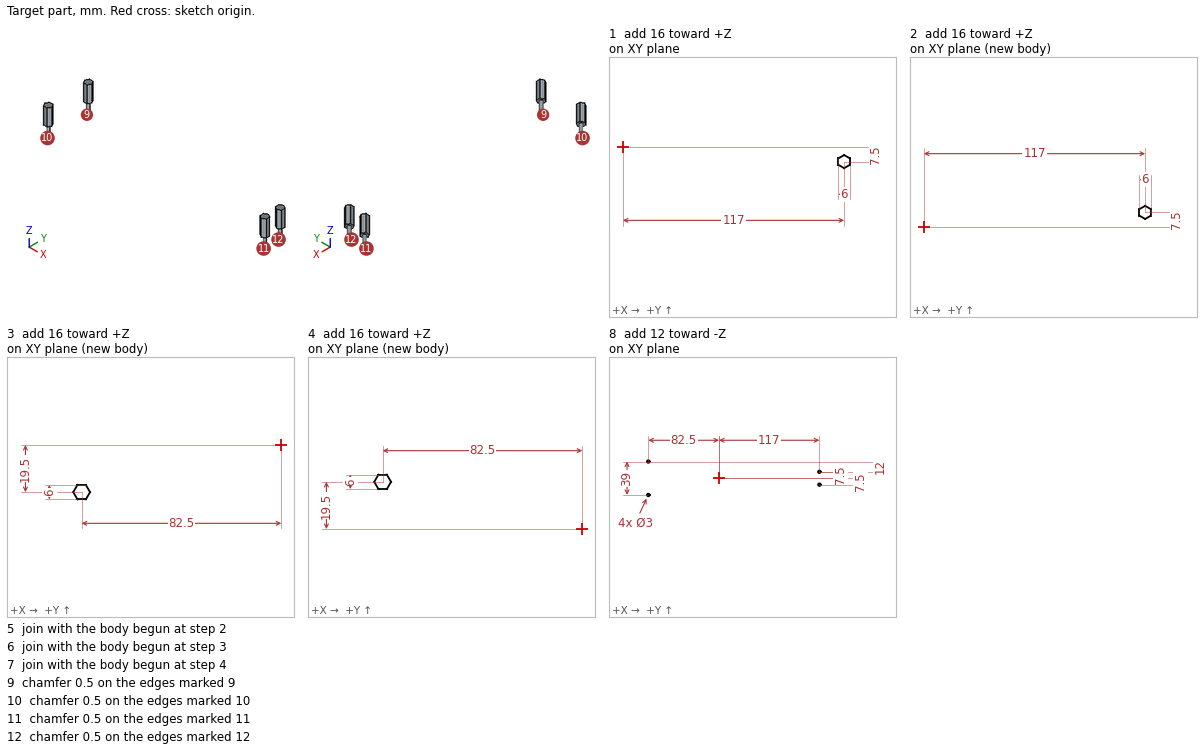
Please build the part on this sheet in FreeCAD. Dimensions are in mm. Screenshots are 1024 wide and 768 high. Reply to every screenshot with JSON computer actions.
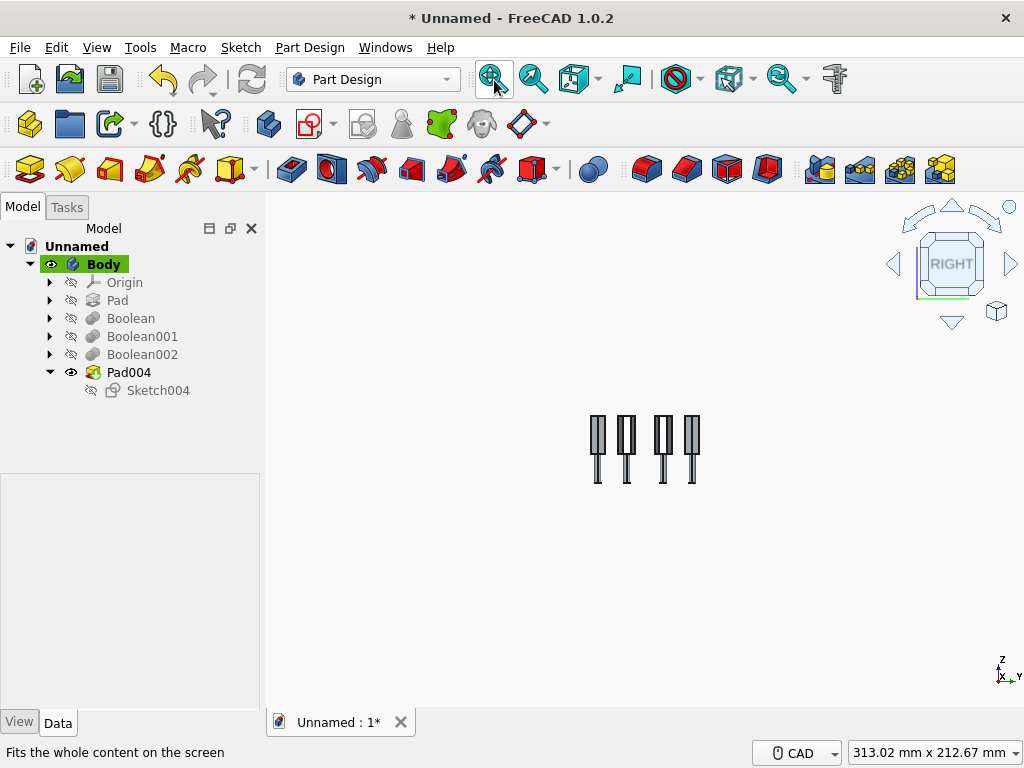
{"action": "left_click", "coordinate": [494, 80]}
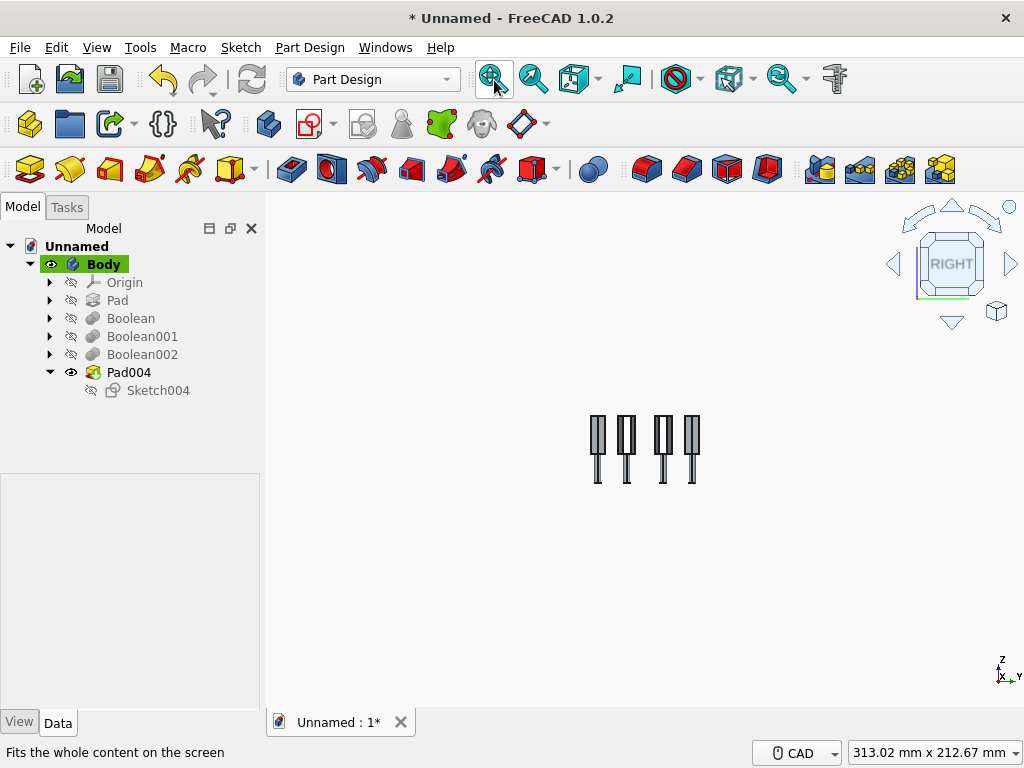
{"action": "key", "text": "5"}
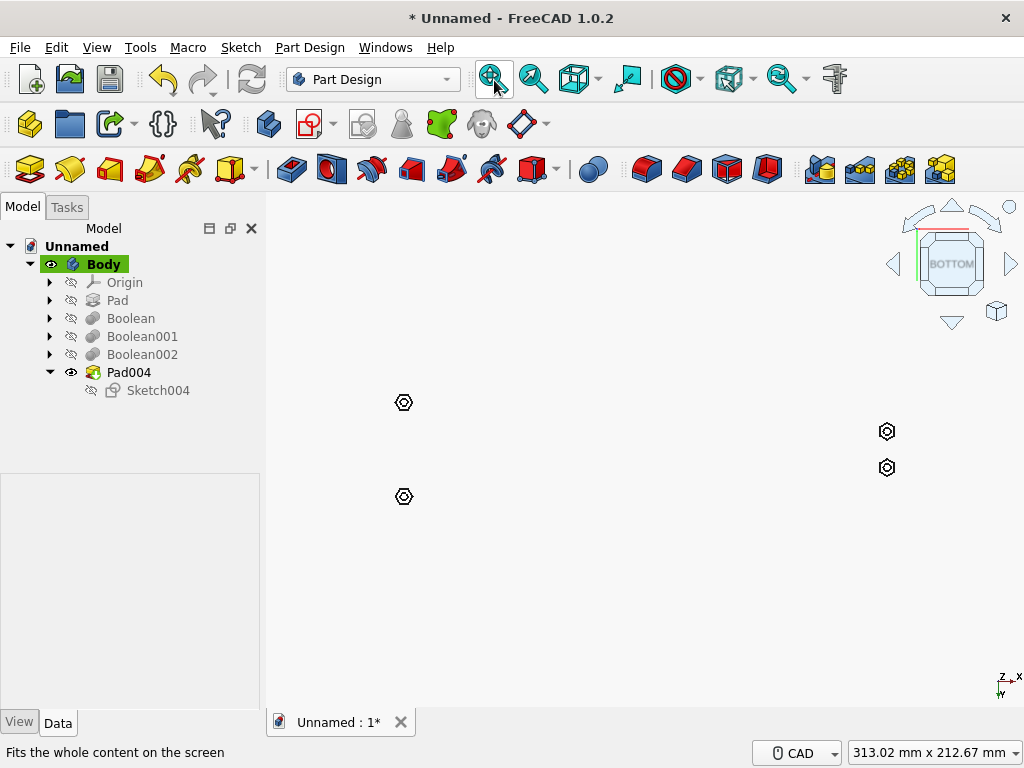
{"action": "left_click", "coordinate": [400, 496]}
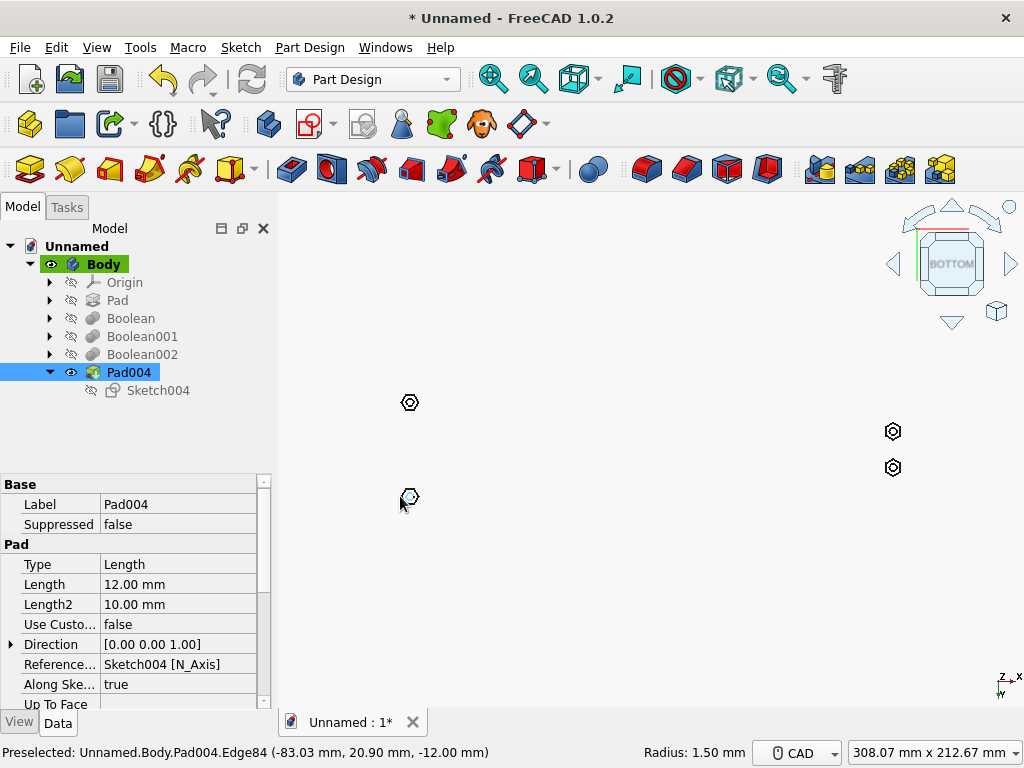
{"action": "left_click", "coordinate": [688, 170]}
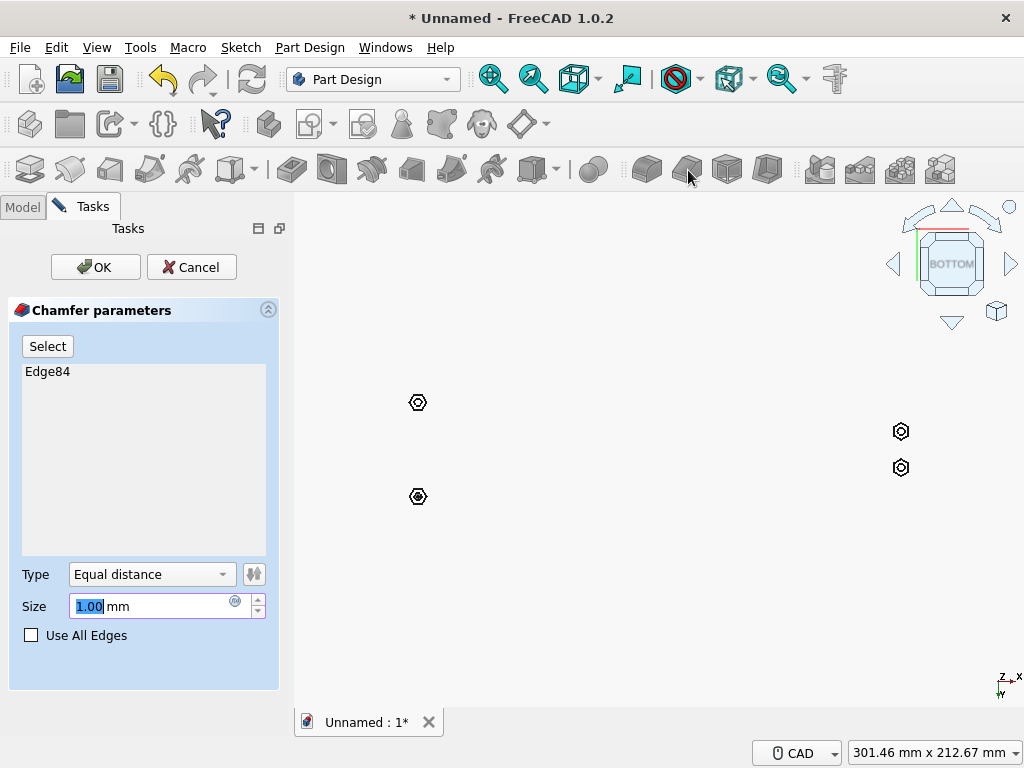
{"action": "type", "text": "0.5"}
{"action": "key", "text": "Tab"}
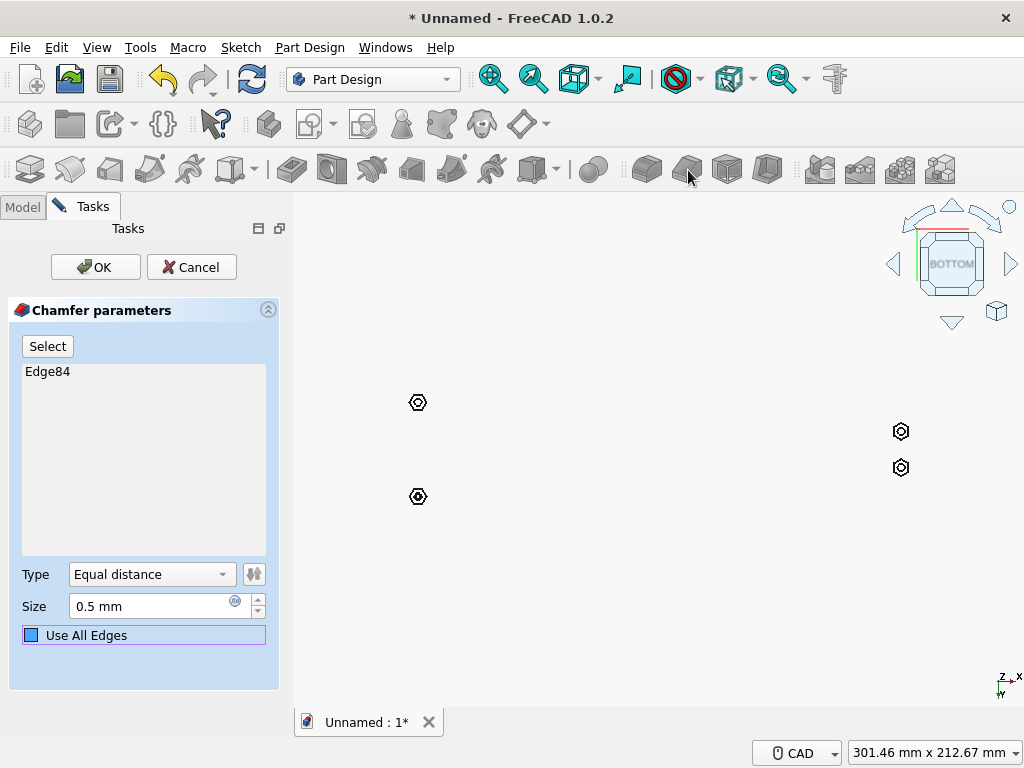
{"action": "left_click", "coordinate": [96, 267]}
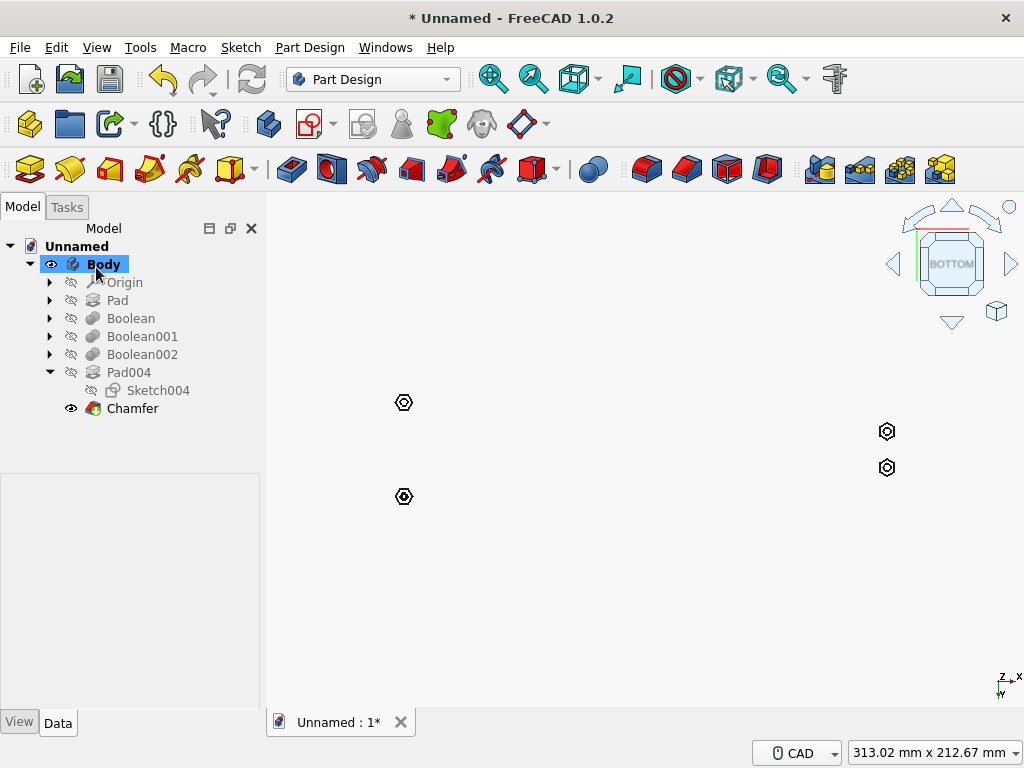
{"action": "left_click", "coordinate": [400, 401]}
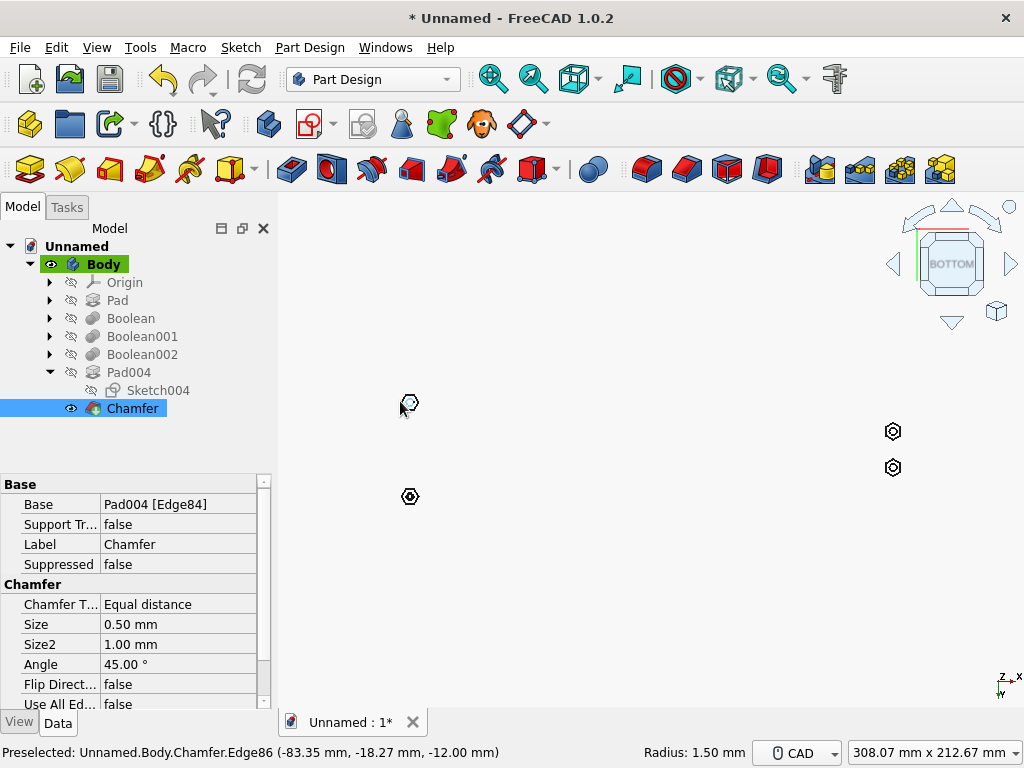
{"action": "left_click", "coordinate": [688, 170]}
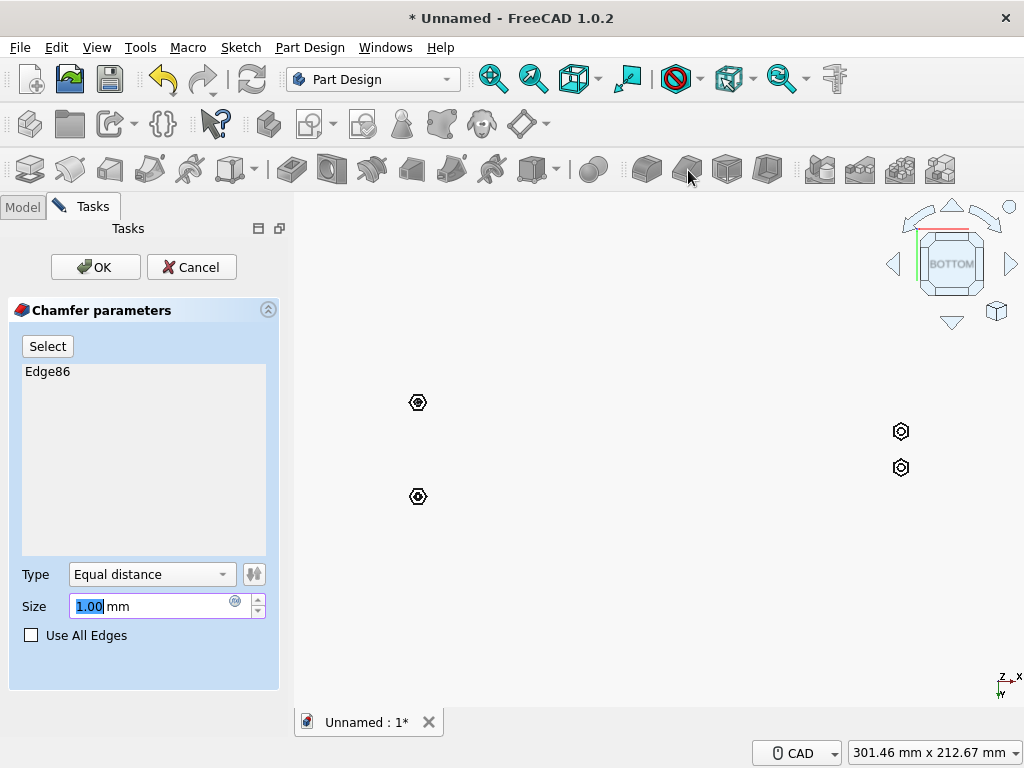
{"action": "type", "text": "0.5"}
{"action": "key", "text": "Tab"}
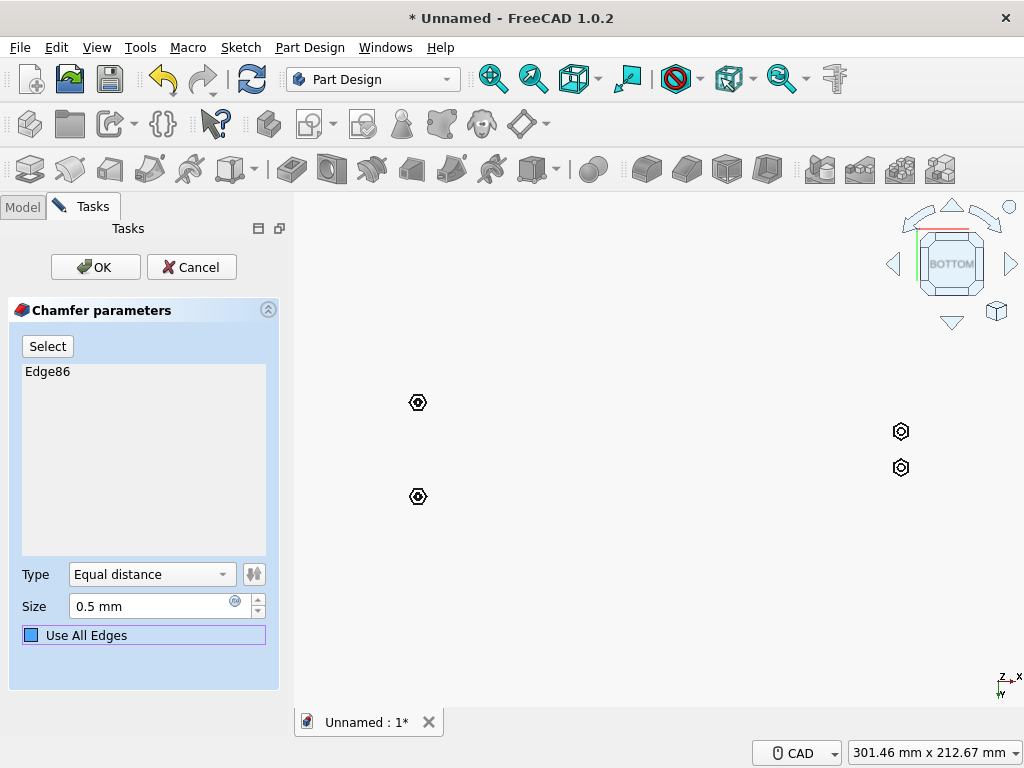
{"action": "left_click", "coordinate": [96, 267]}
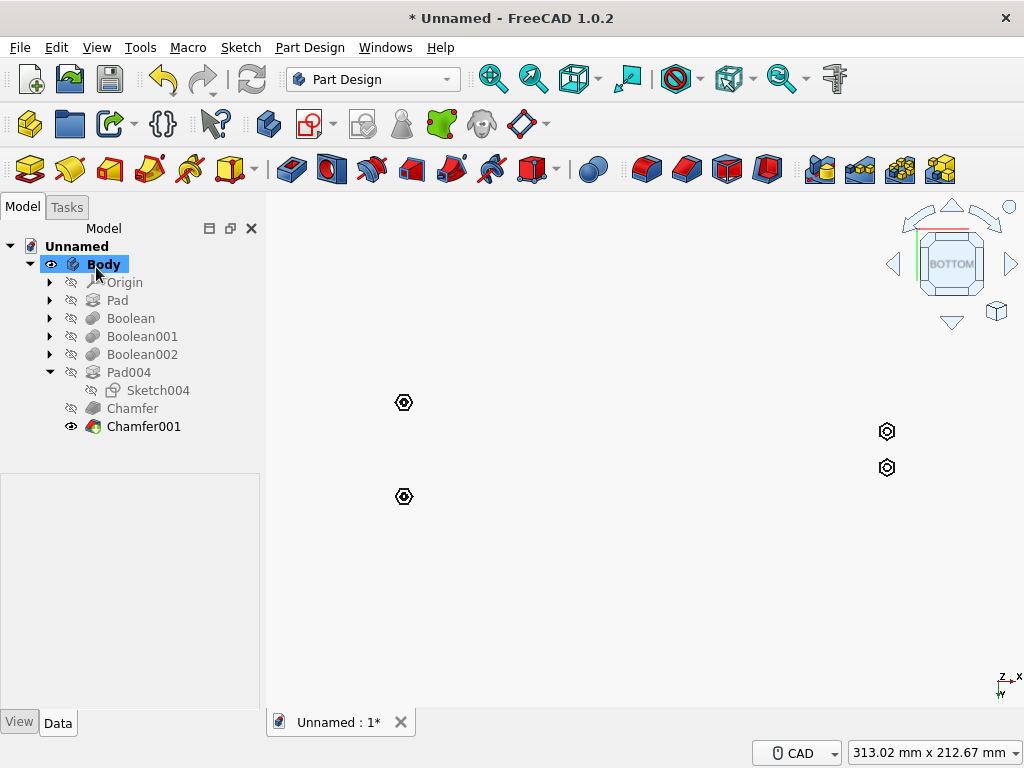
{"action": "left_click", "coordinate": [883, 430]}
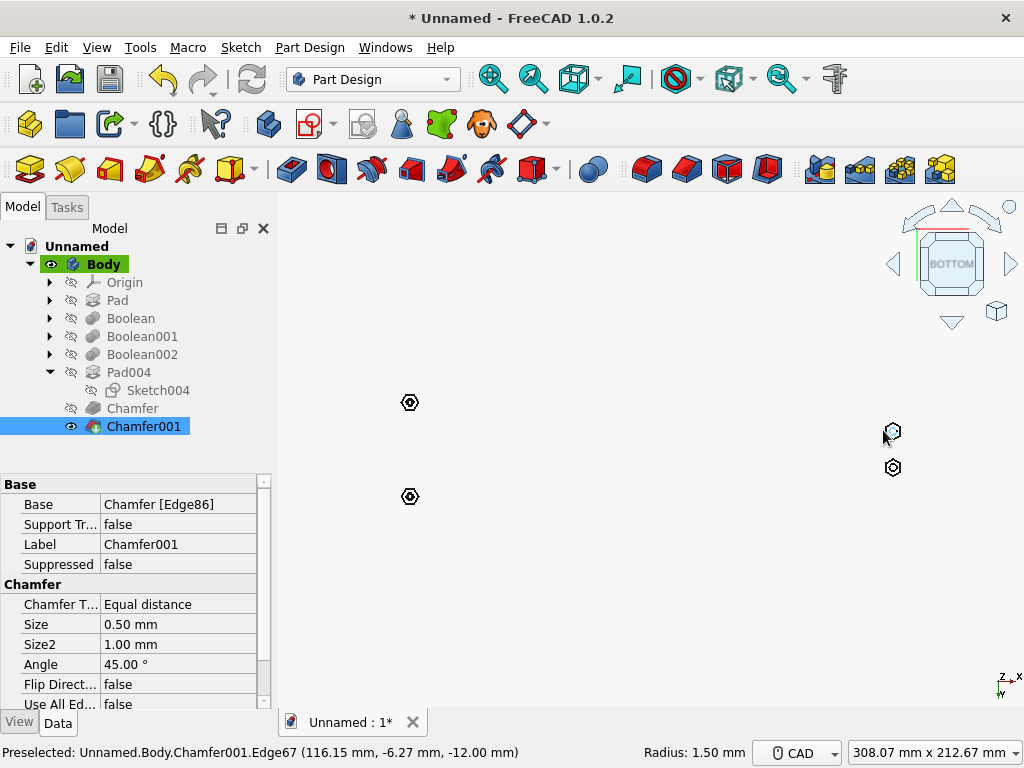
{"action": "left_click", "coordinate": [688, 170]}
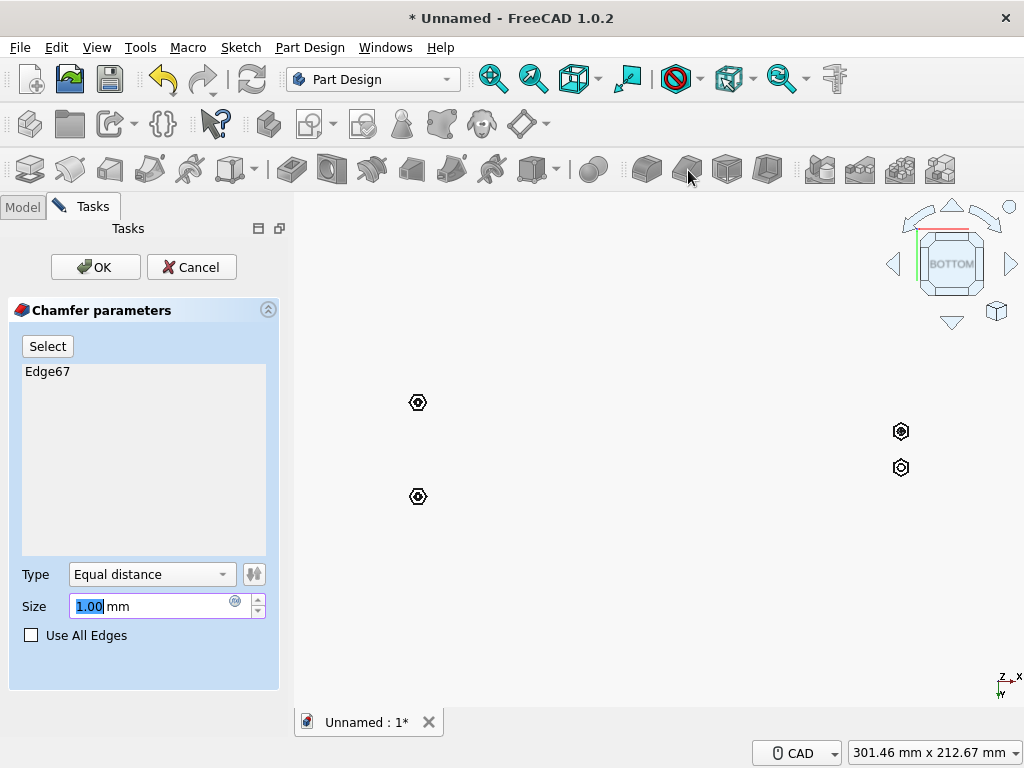
{"action": "type", "text": "0.5"}
{"action": "key", "text": "Tab"}